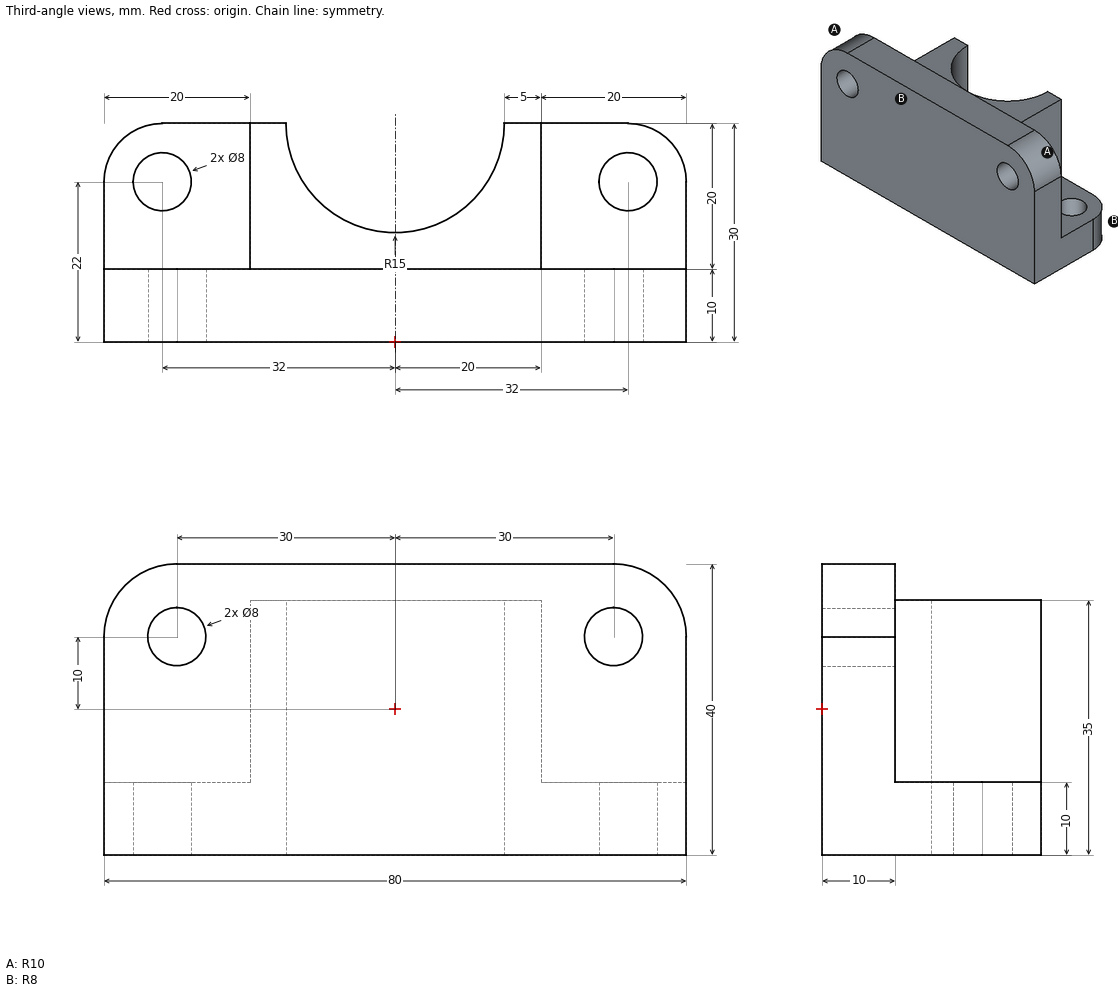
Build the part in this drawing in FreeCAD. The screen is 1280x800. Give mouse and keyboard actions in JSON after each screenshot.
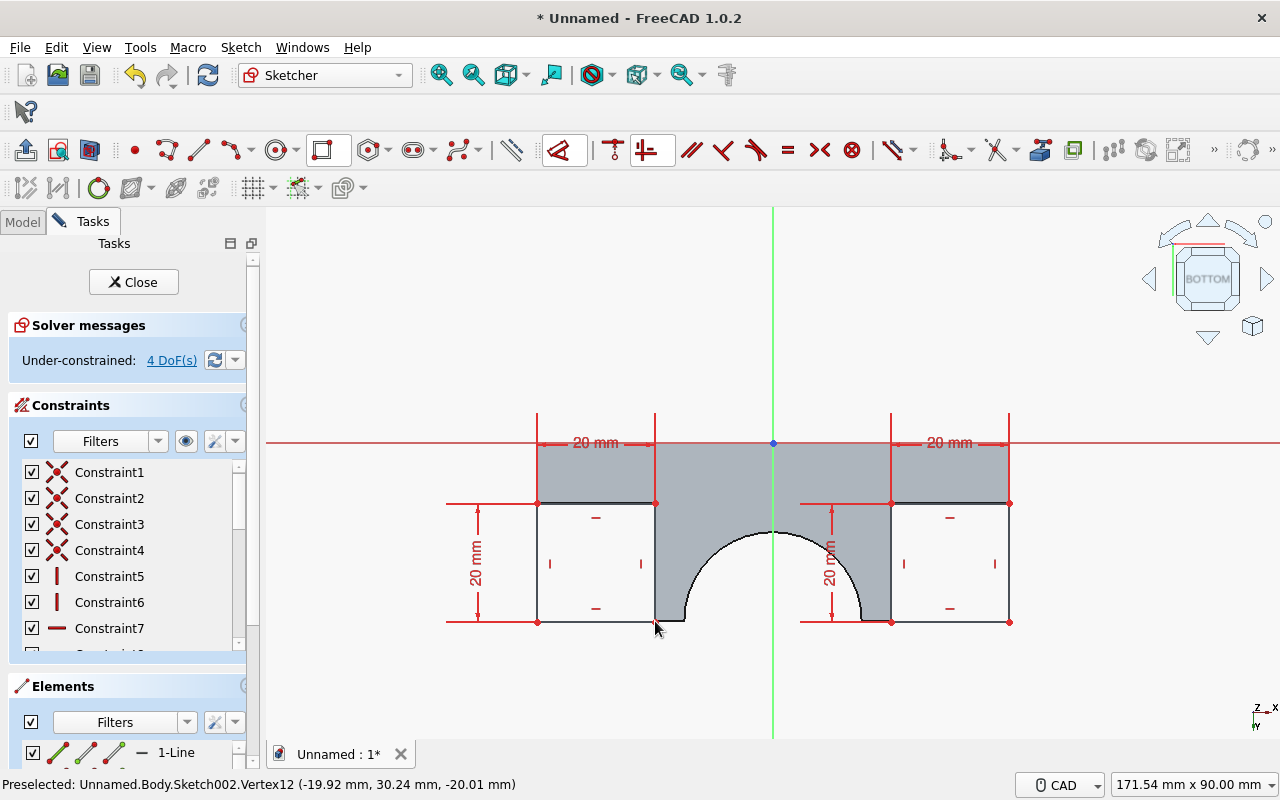
{"action": "left_click", "coordinate": [1009, 504]}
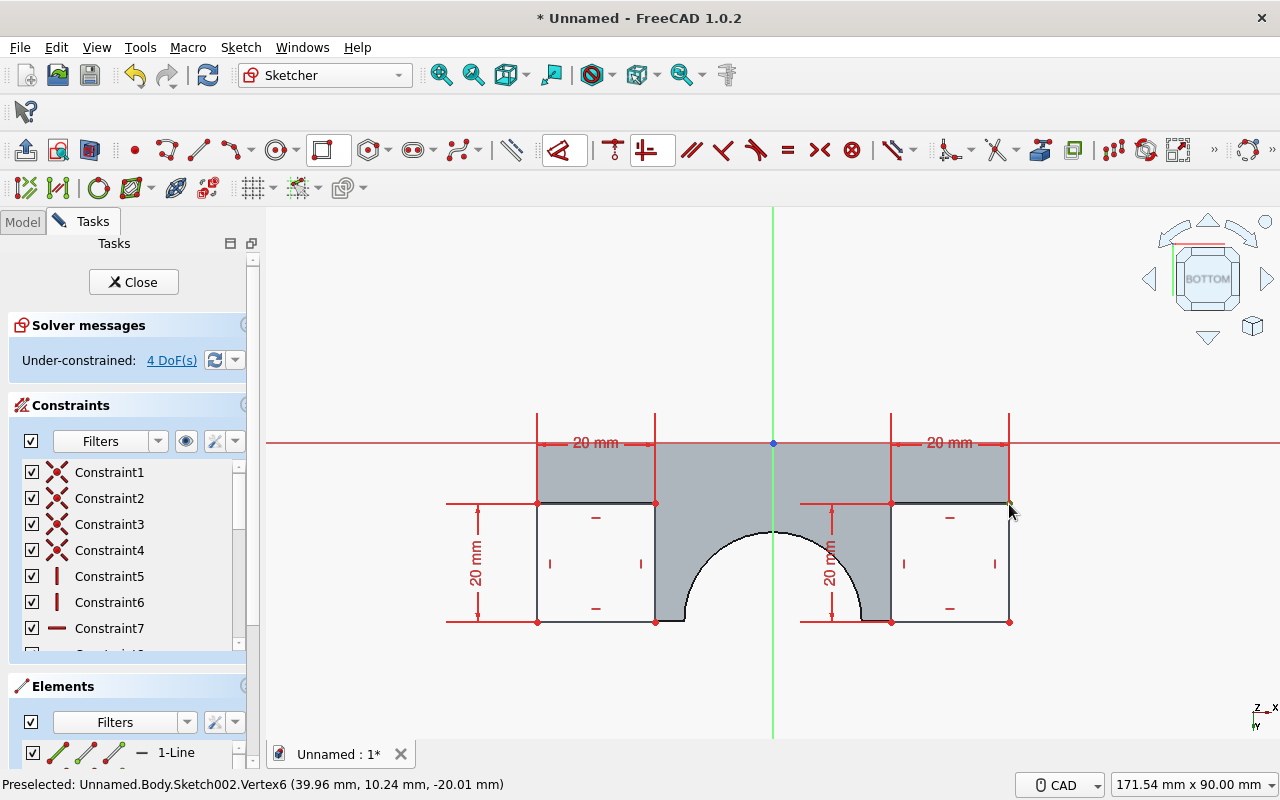
{"action": "left_click", "coordinate": [537, 504]}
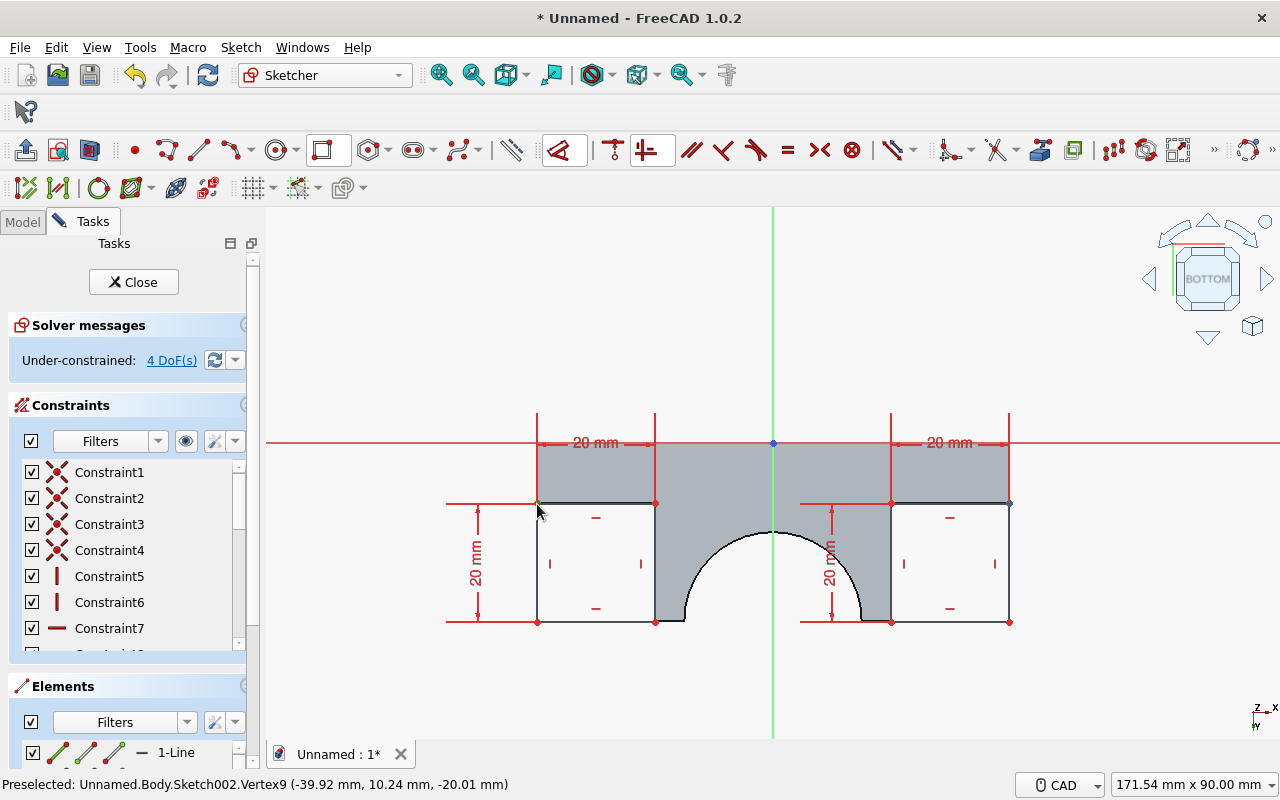
{"action": "left_click", "coordinate": [773, 677]}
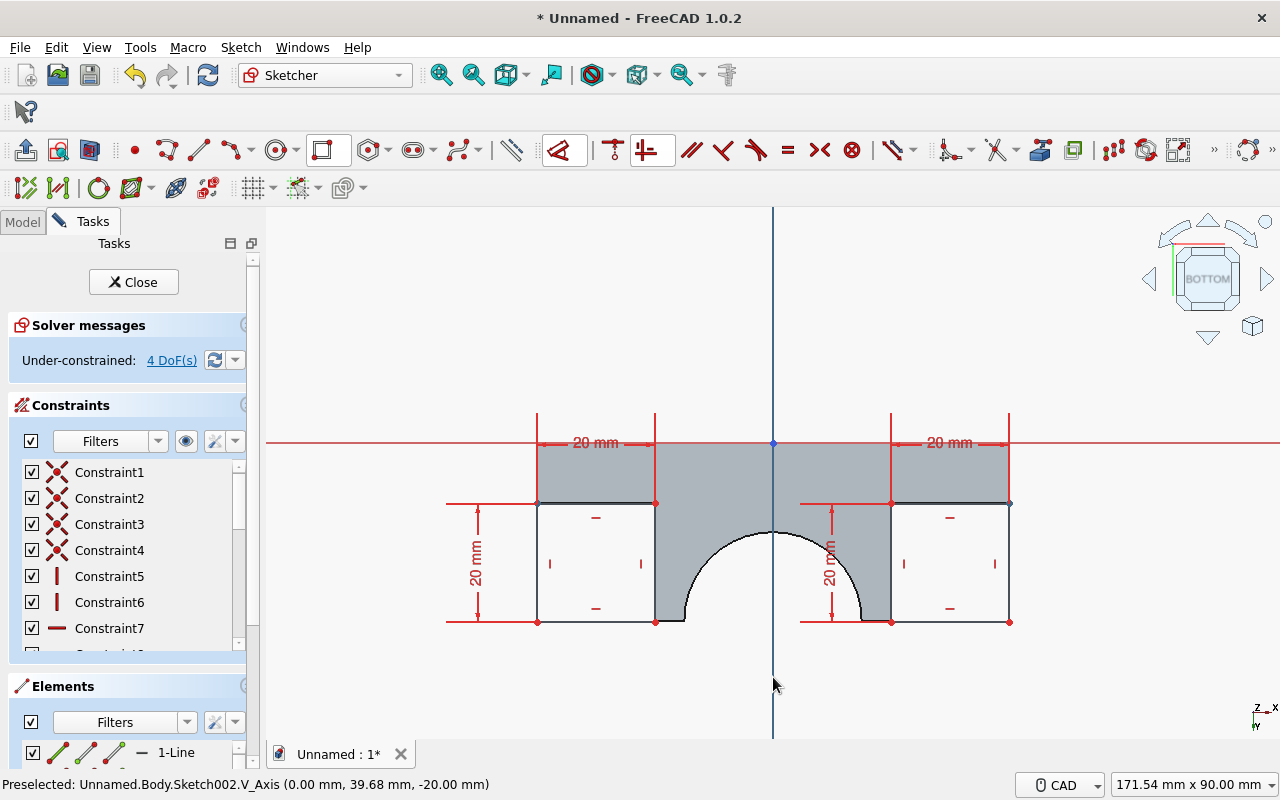
{"action": "left_click", "coordinate": [820, 150]}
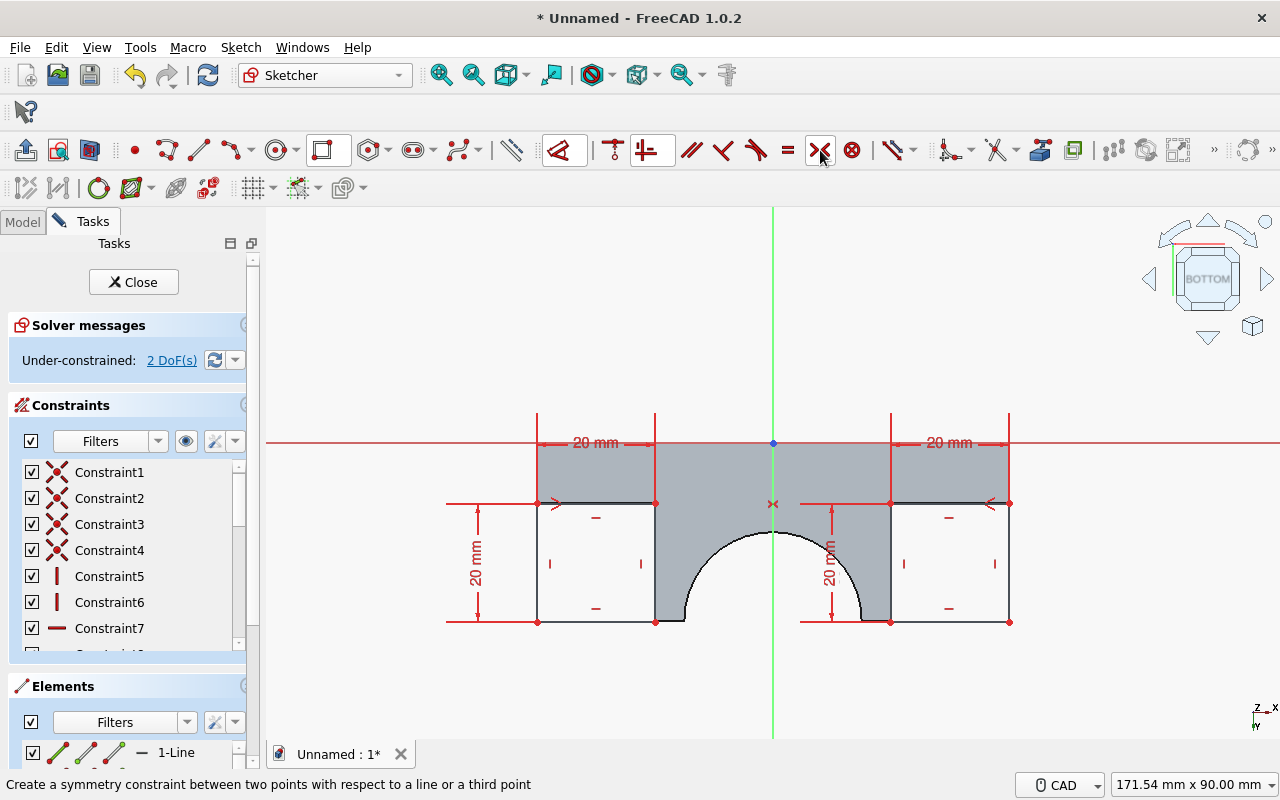
{"action": "left_click", "coordinate": [891, 504]}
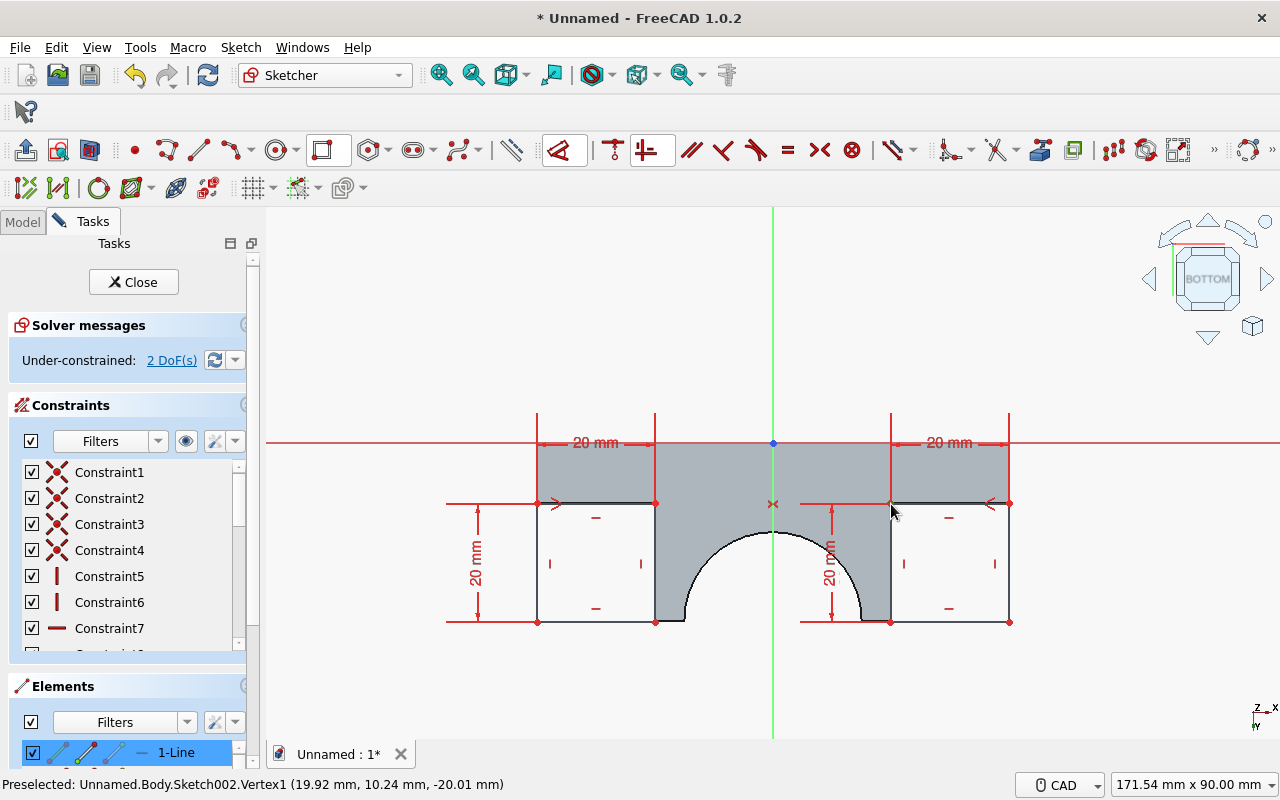
{"action": "key", "text": "l"}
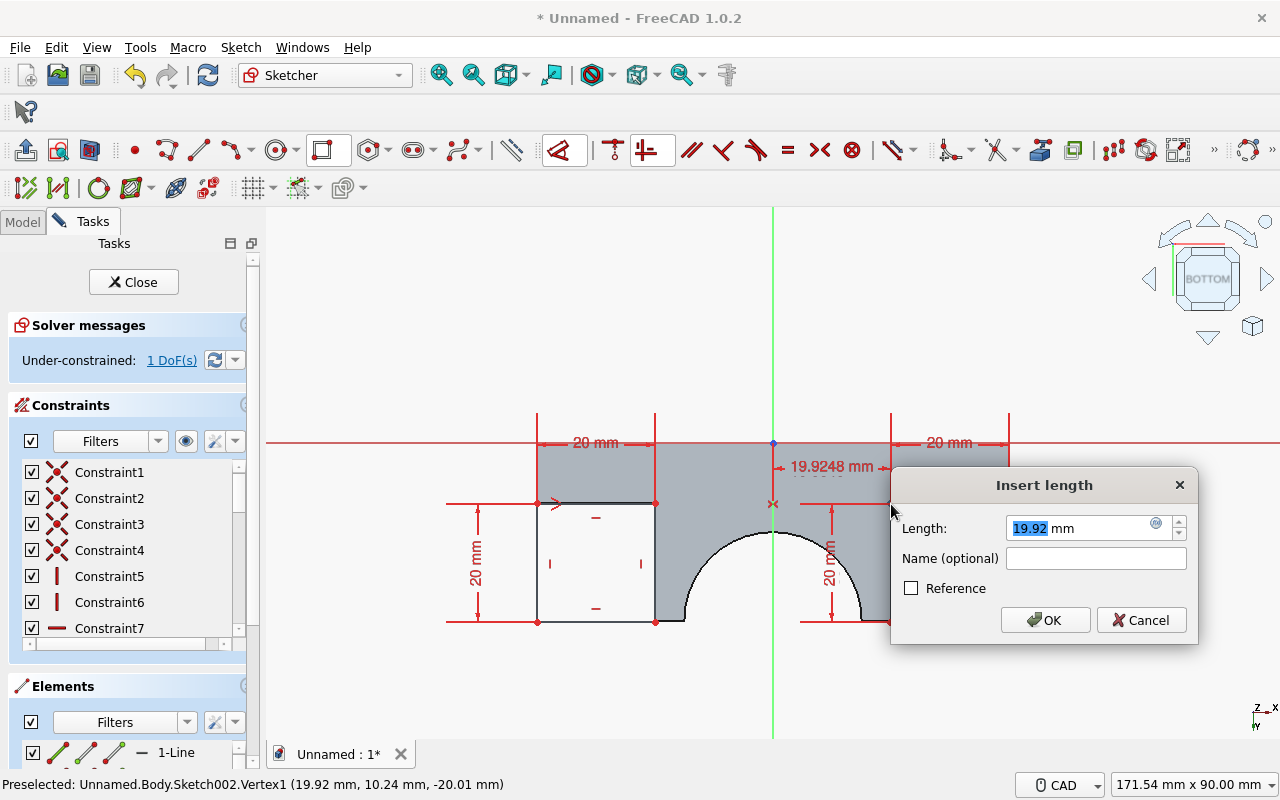
{"action": "type", "text": "20"}
{"action": "key", "text": "Return"}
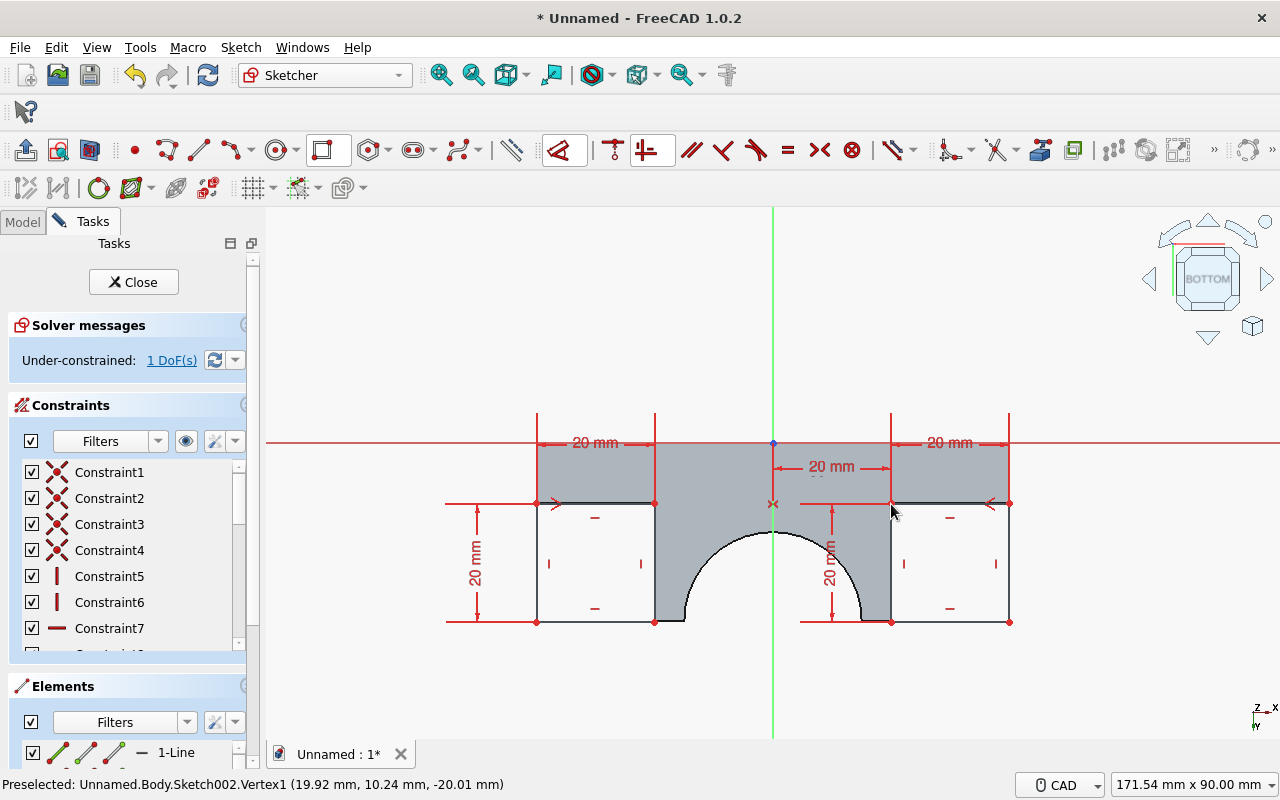
{"action": "left_click", "coordinate": [891, 504]}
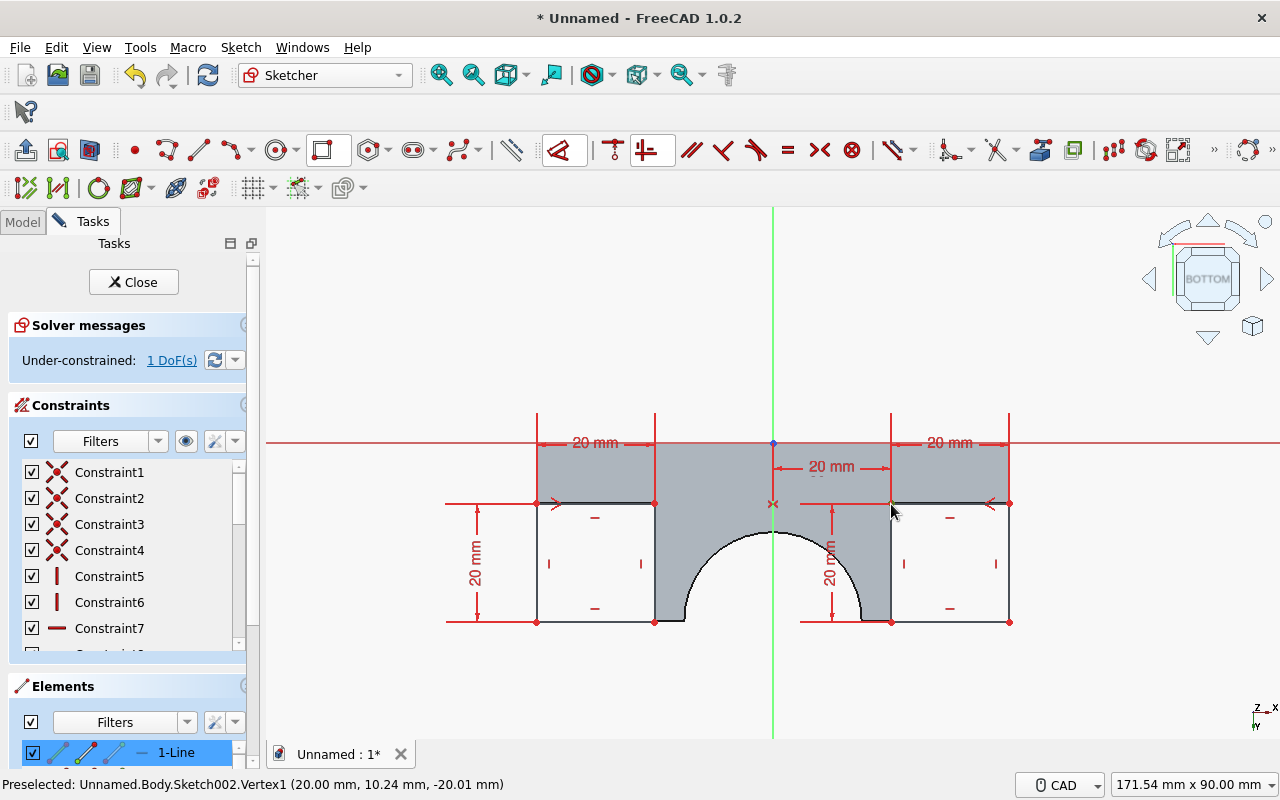
{"action": "key", "text": "i"}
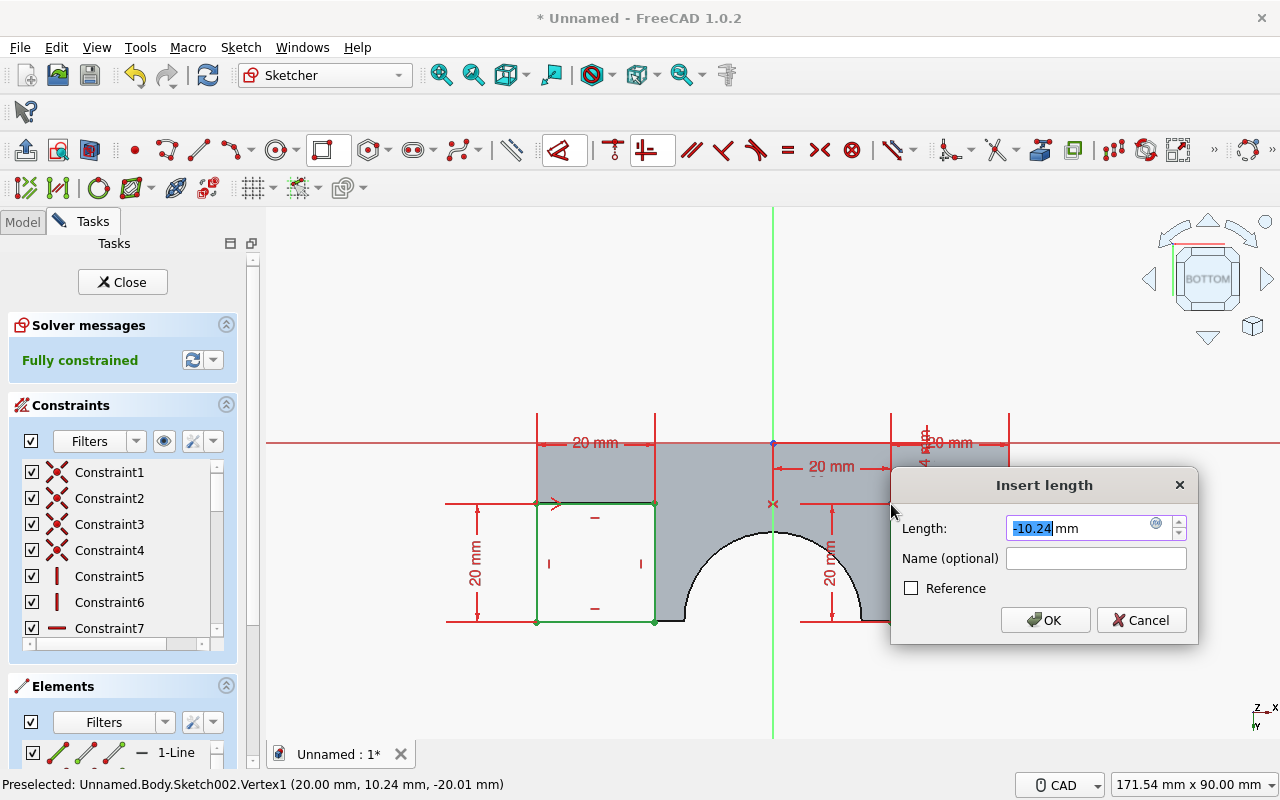
{"action": "type", "text": "-10"}
{"action": "key", "text": "Return"}